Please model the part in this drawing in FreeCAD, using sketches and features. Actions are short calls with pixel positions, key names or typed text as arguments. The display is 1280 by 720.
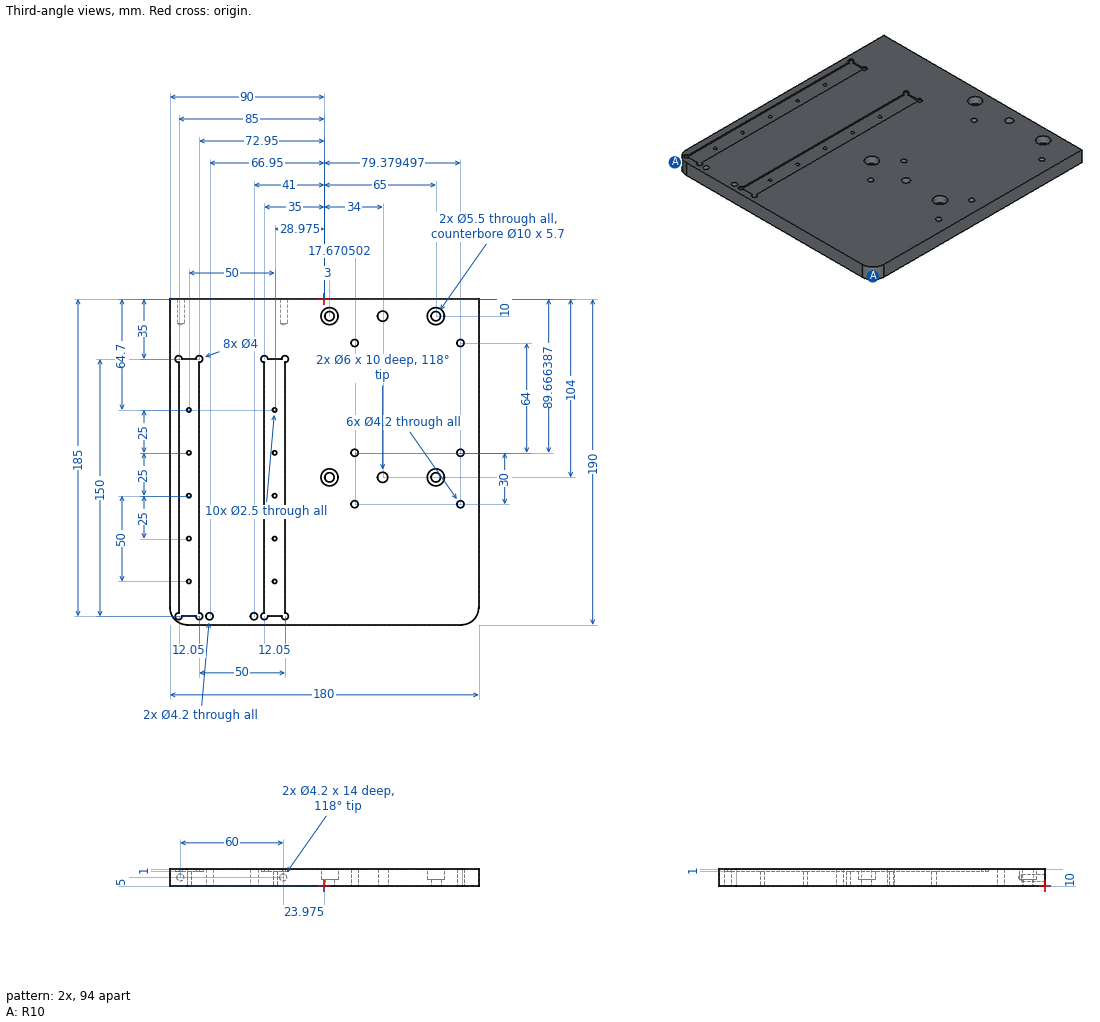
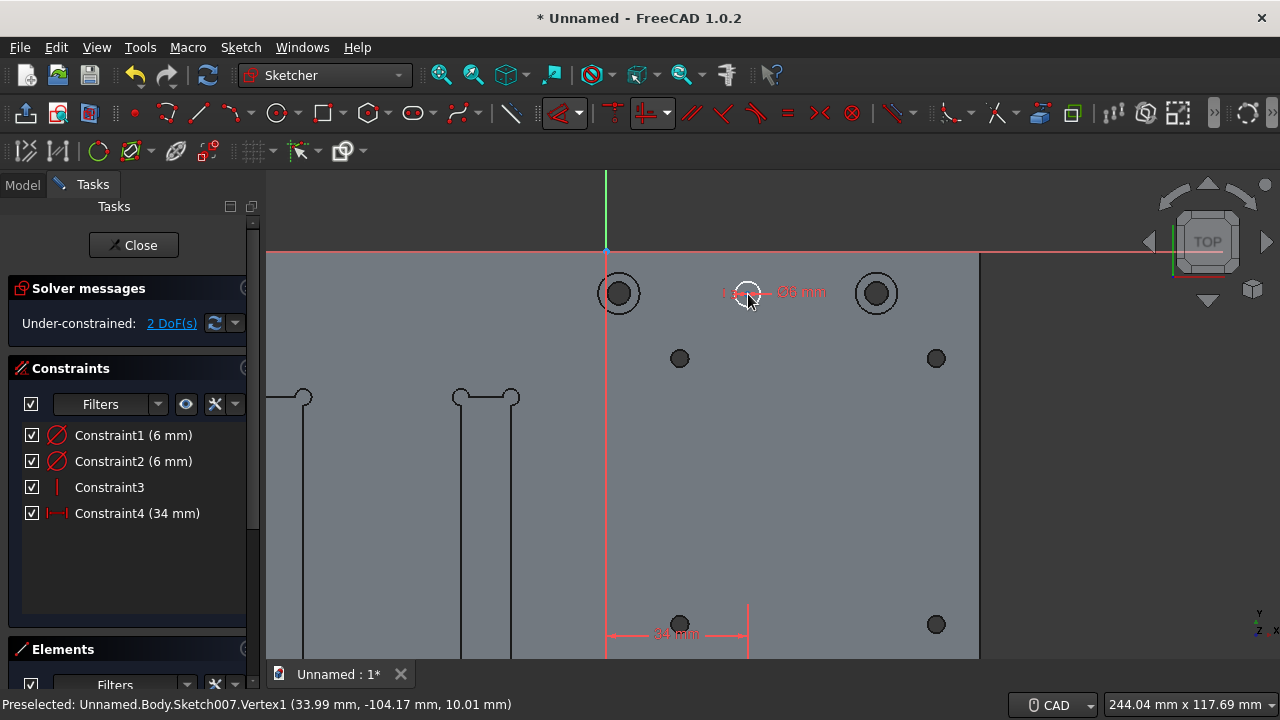
click(748, 294)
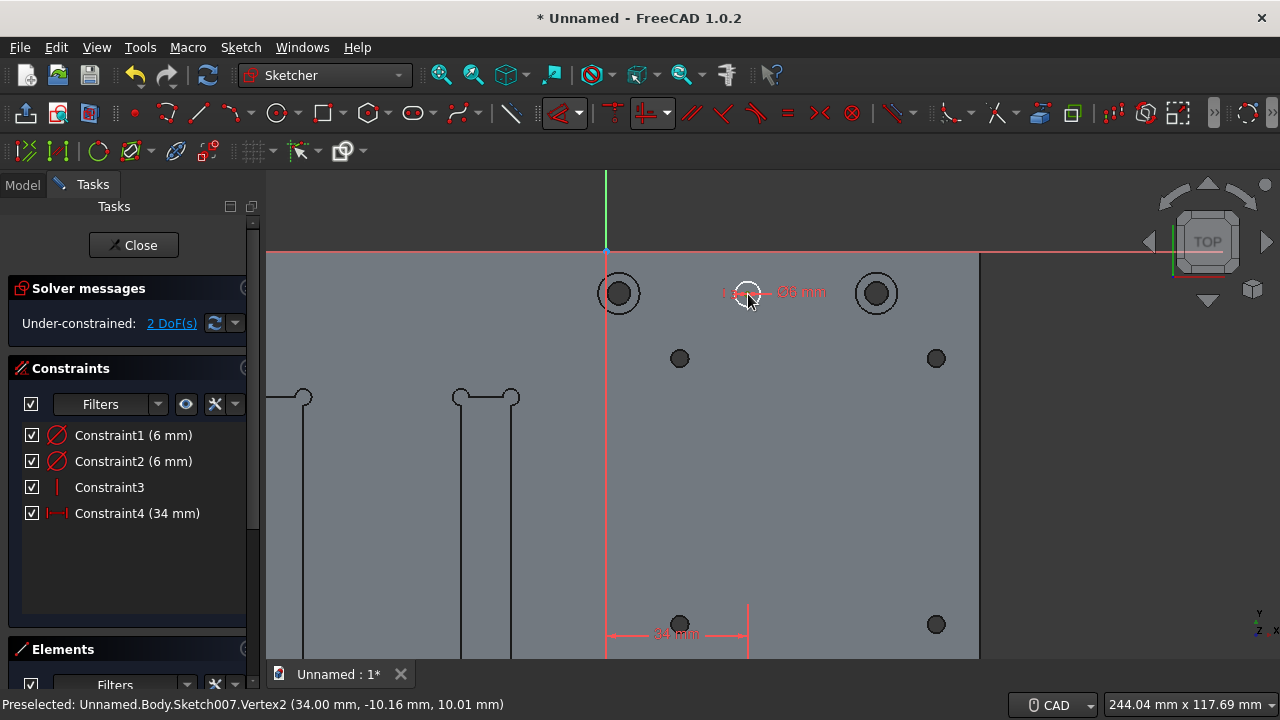
click(582, 114)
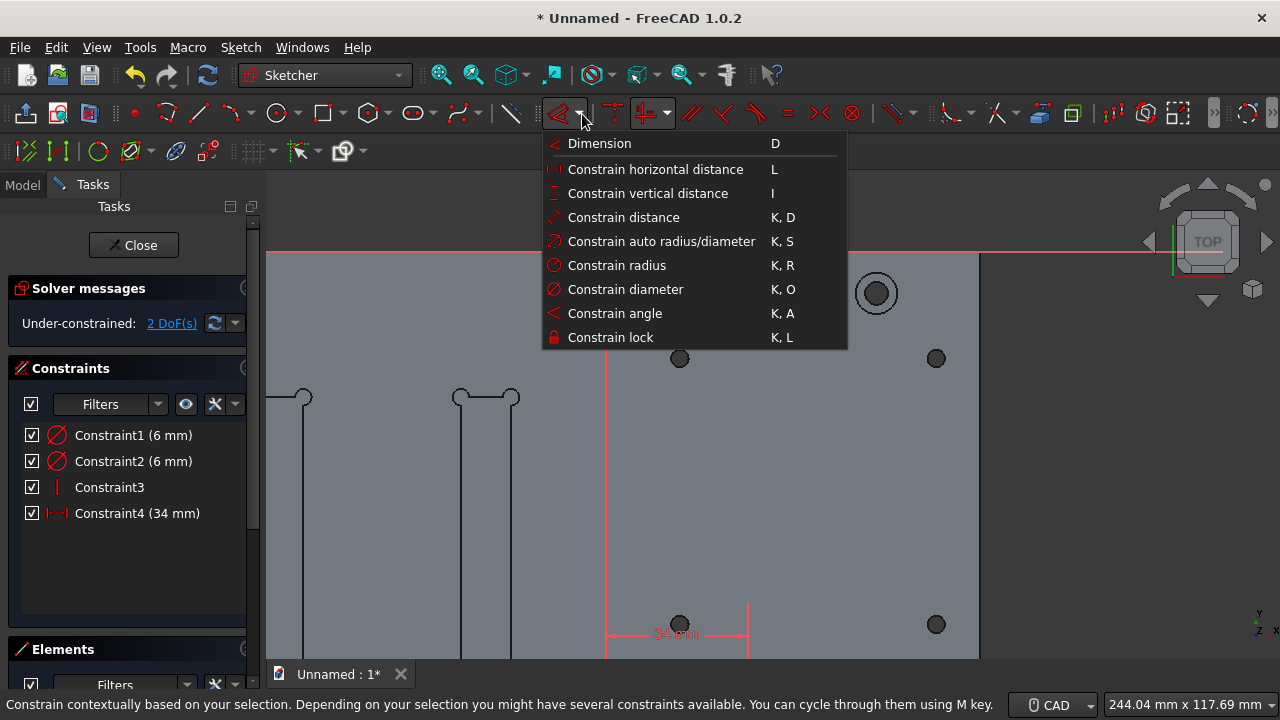
click(695, 193)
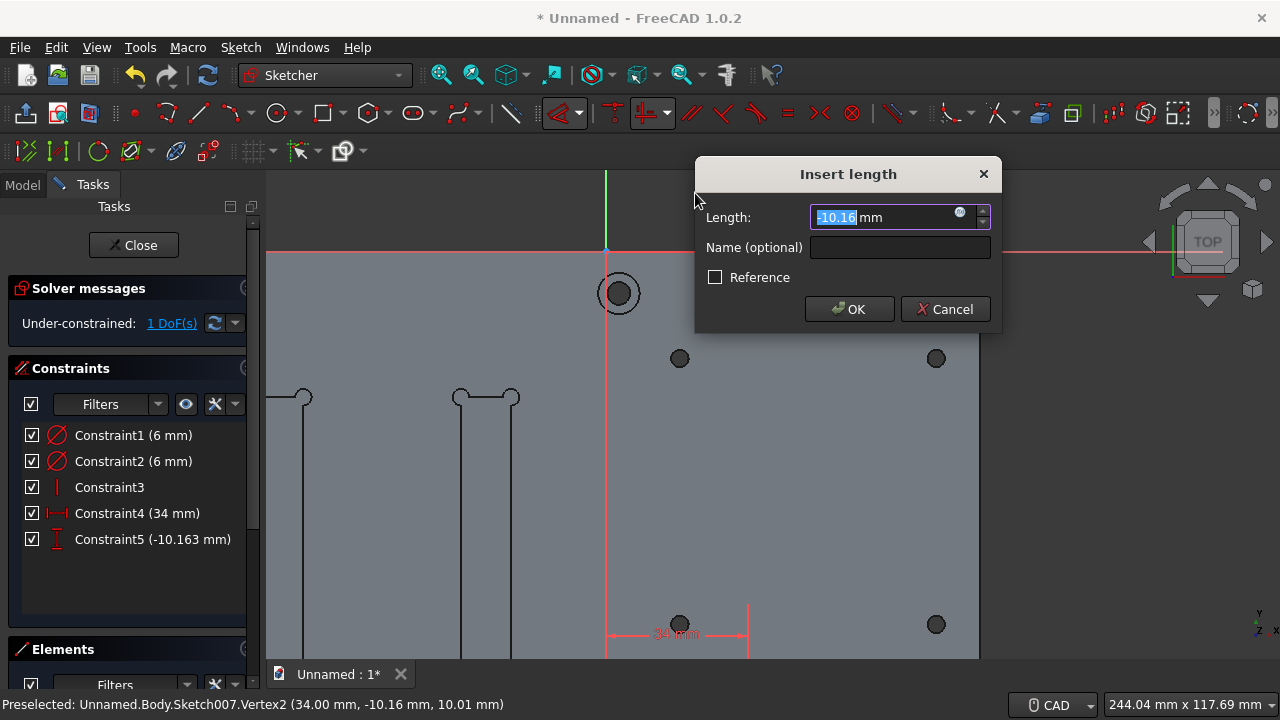
text(-10)
key(Return)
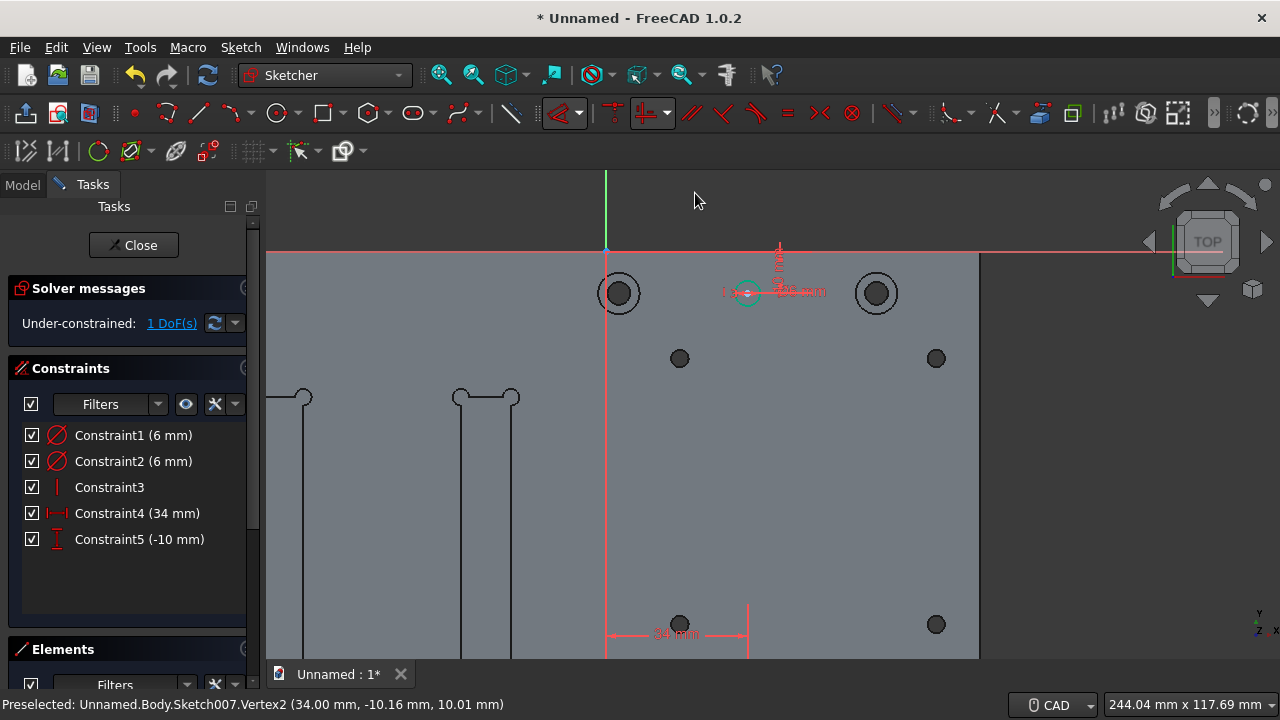
scroll(748, 293, down, 2)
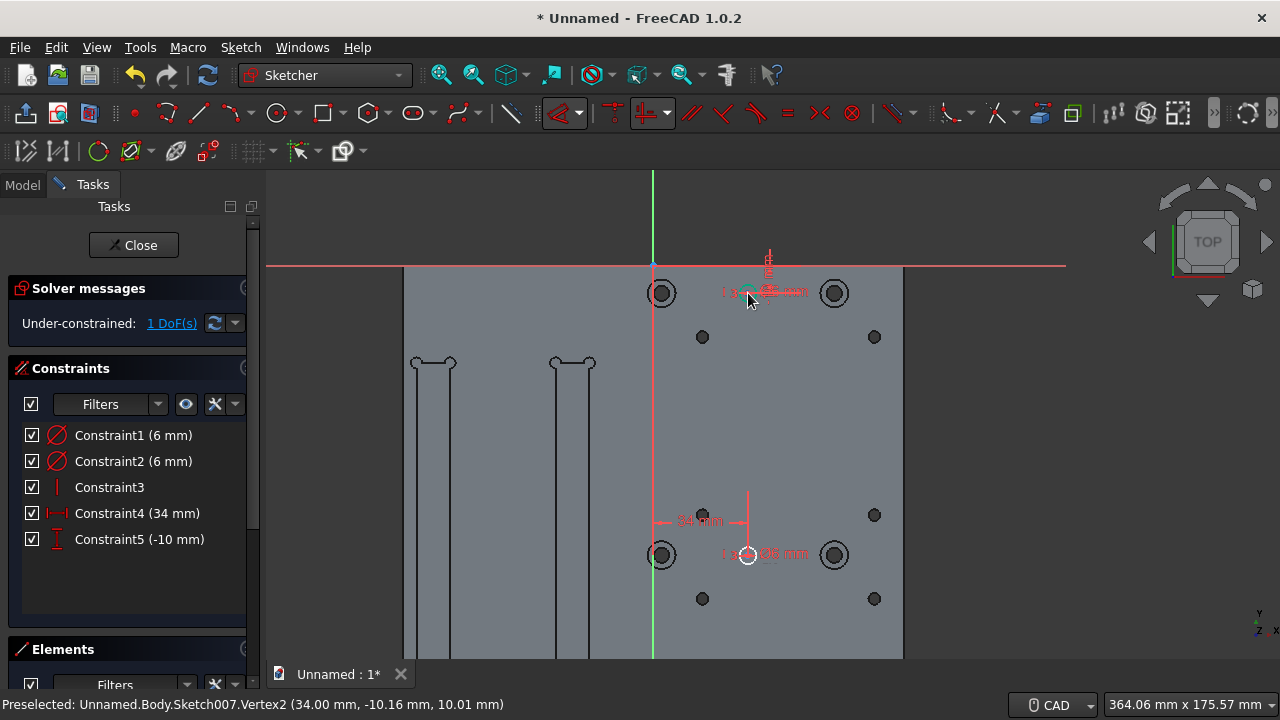
click(748, 556)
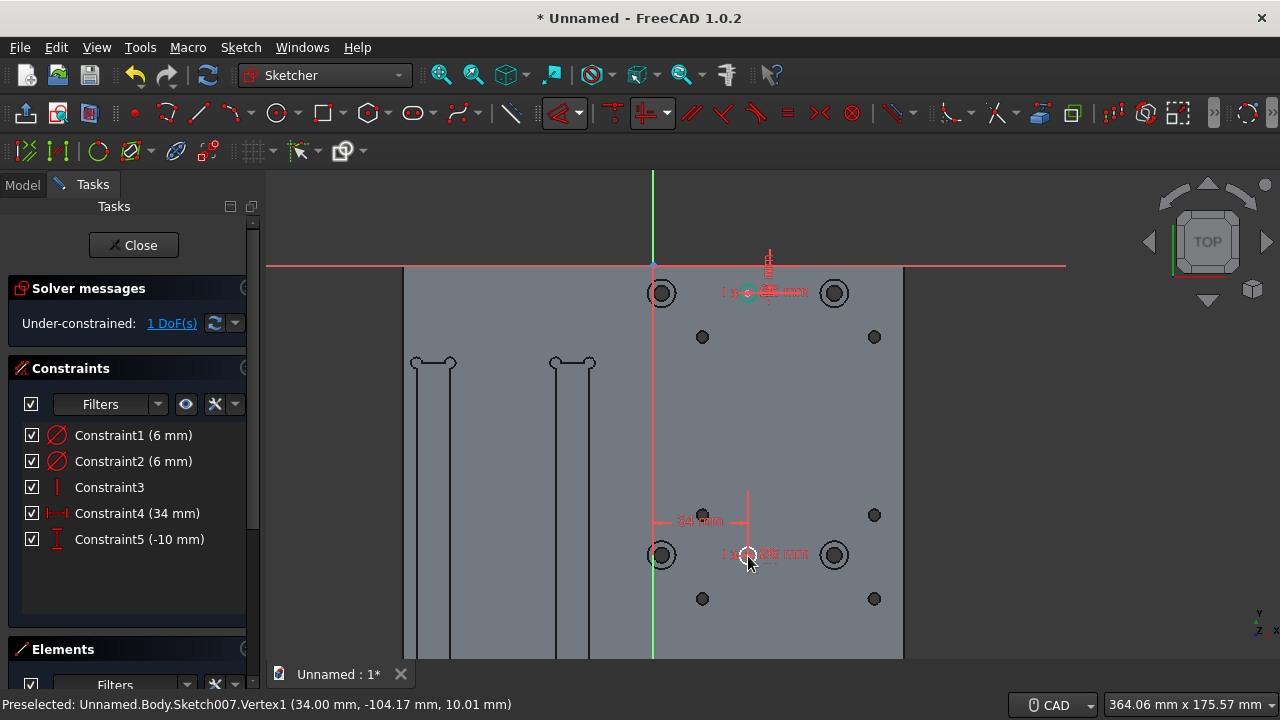
key(i)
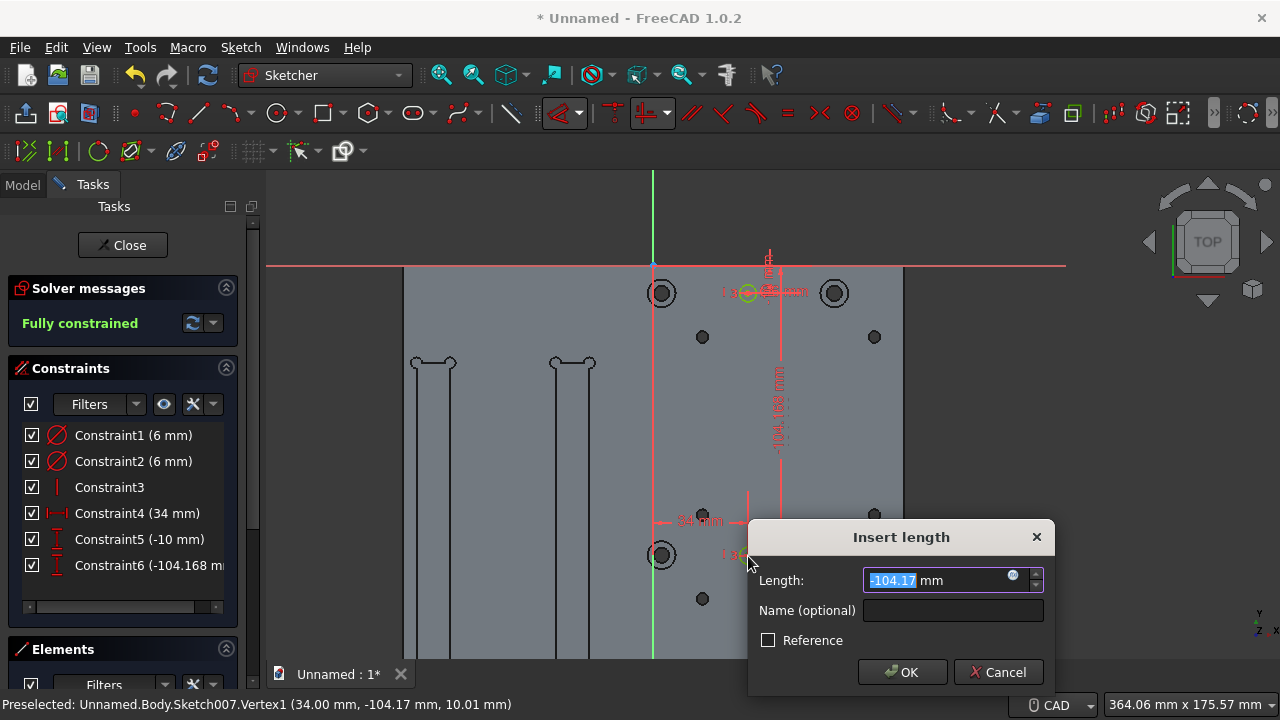
text(-104)
key(Return)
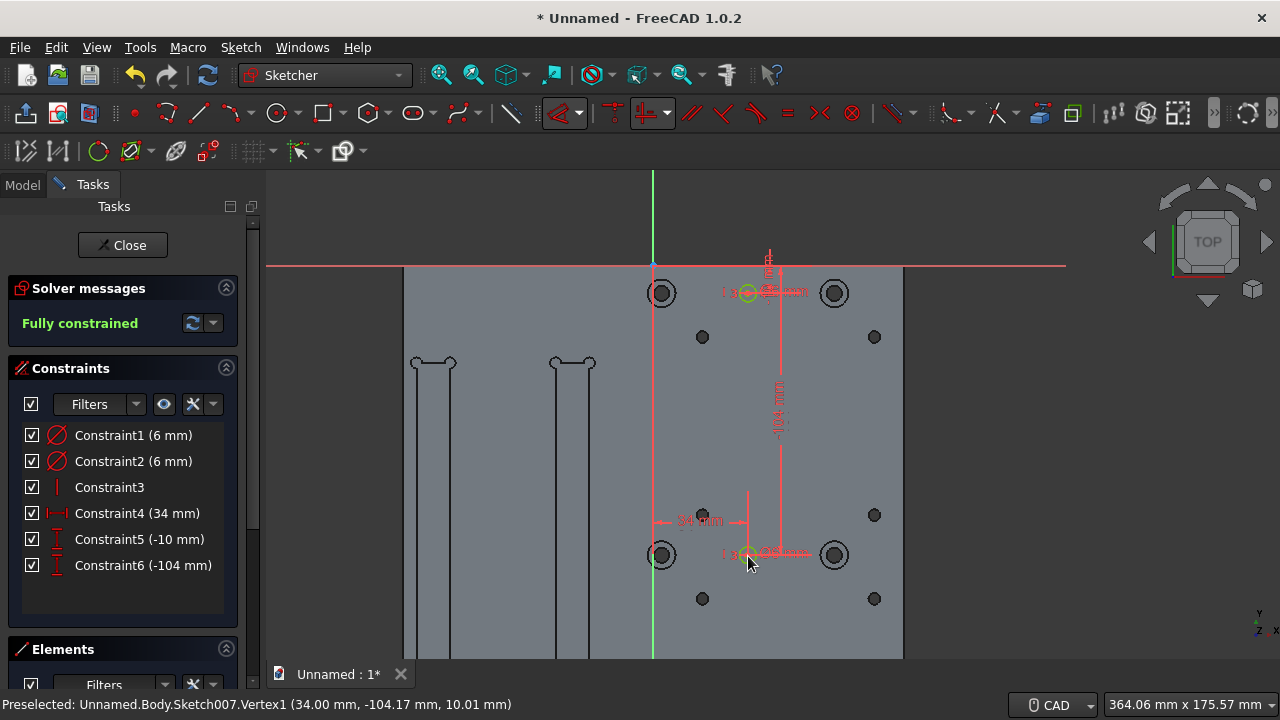
click(123, 245)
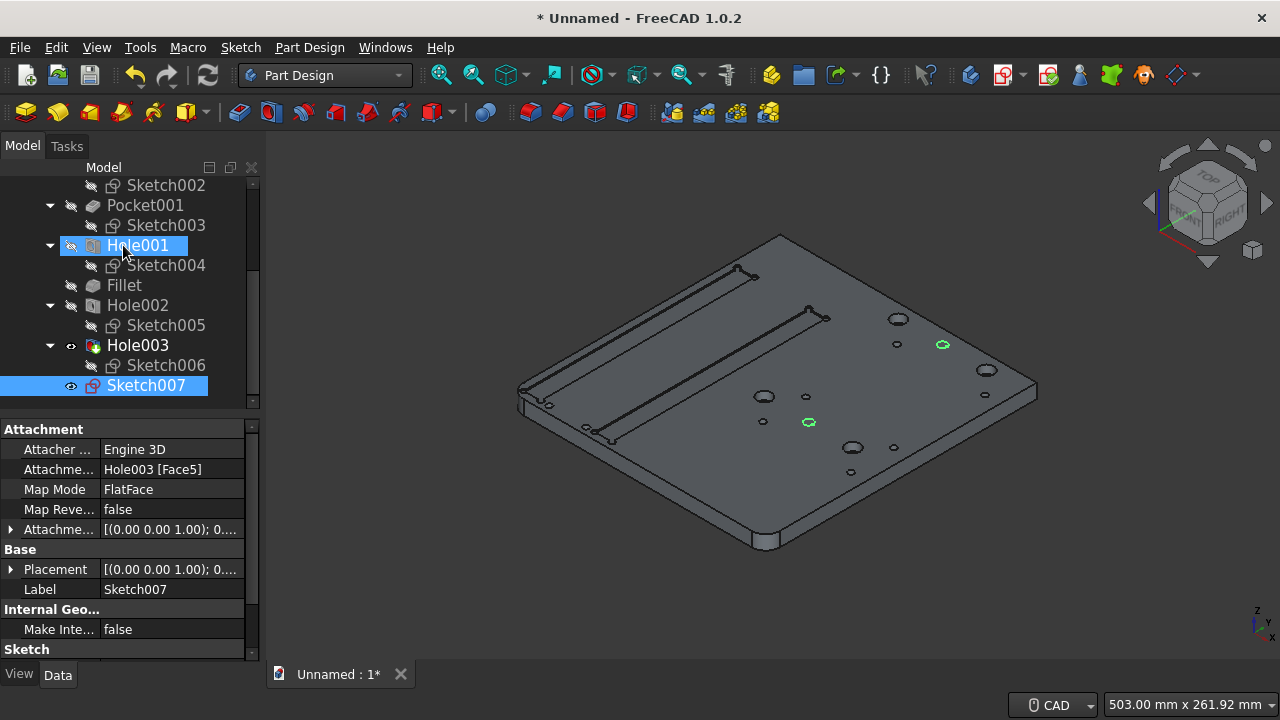
click(272, 112)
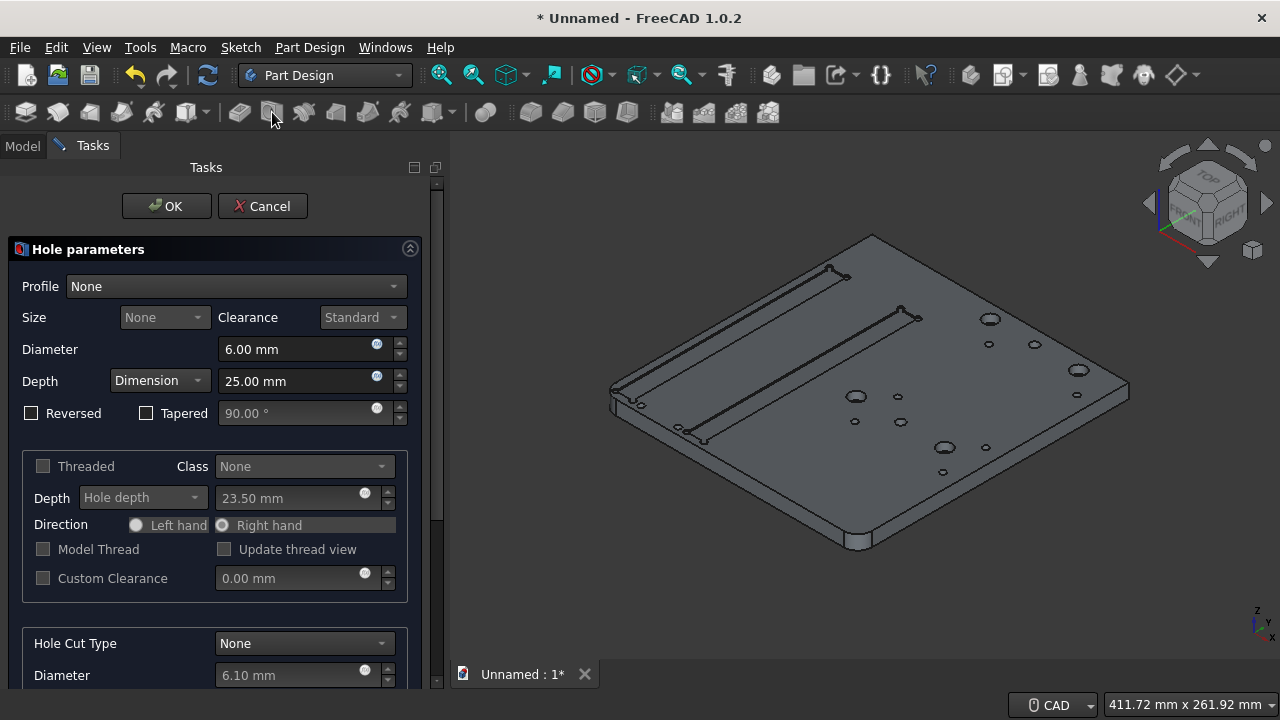
triple_click(305, 349)